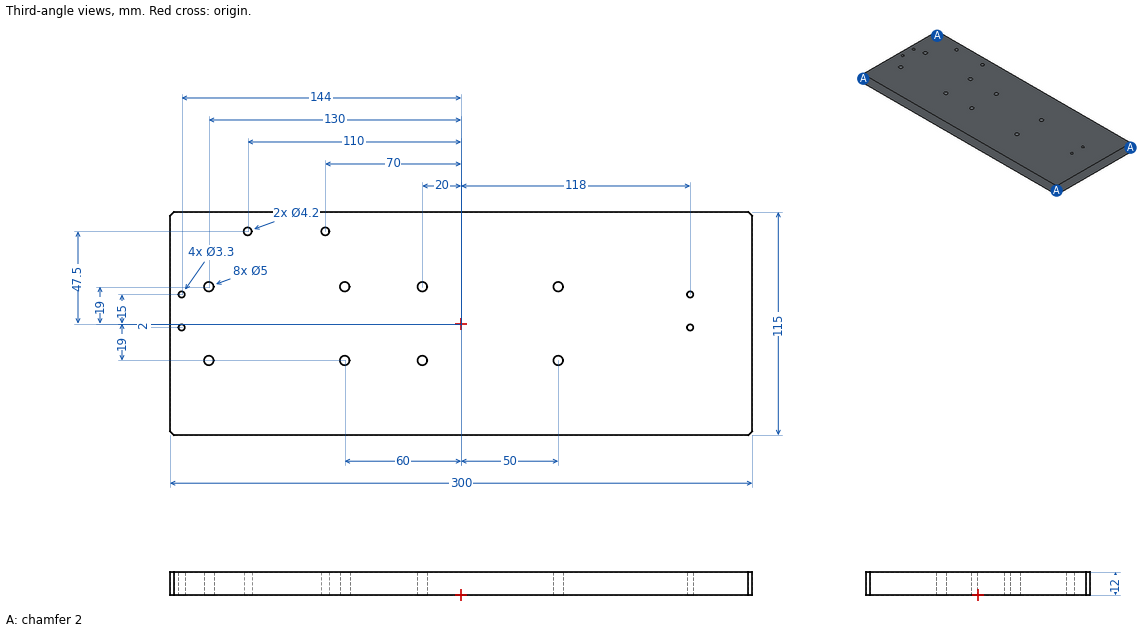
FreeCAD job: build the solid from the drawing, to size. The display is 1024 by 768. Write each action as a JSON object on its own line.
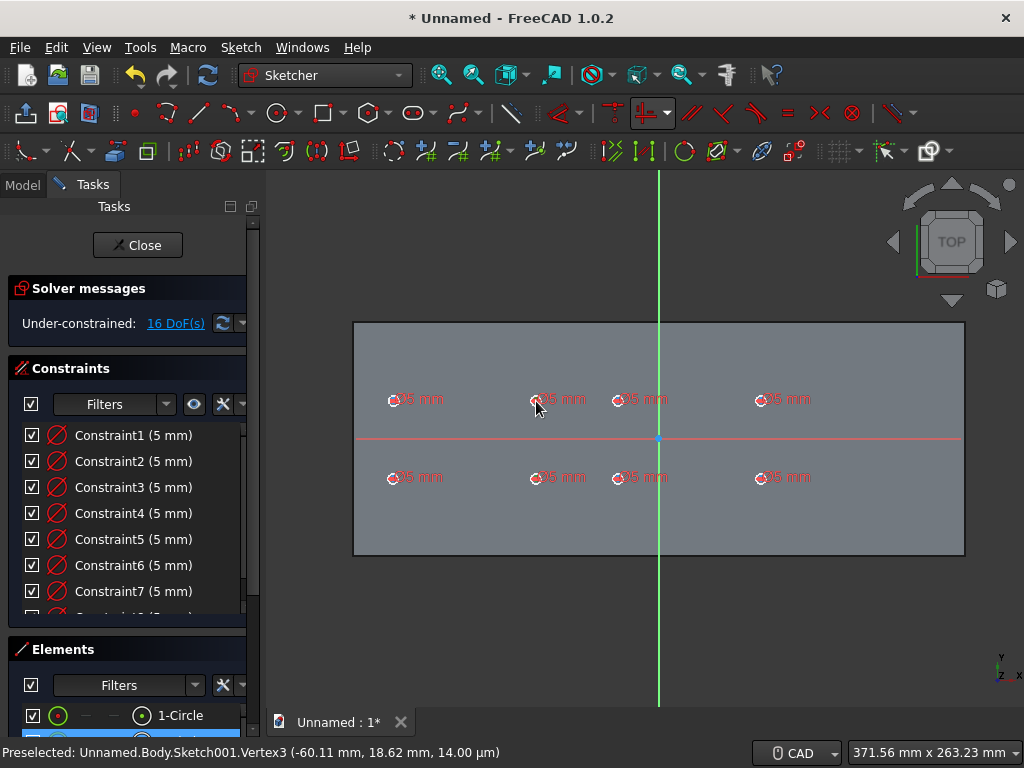
{"action": "left_click", "coordinate": [670, 114]}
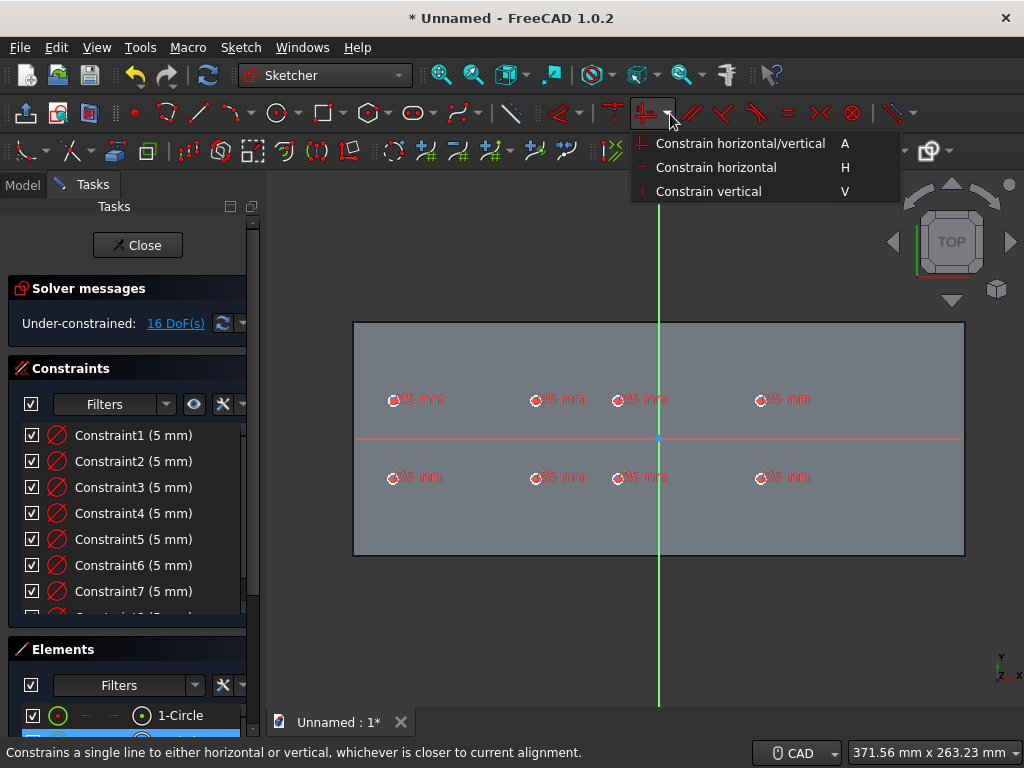
{"action": "left_click", "coordinate": [766, 191]}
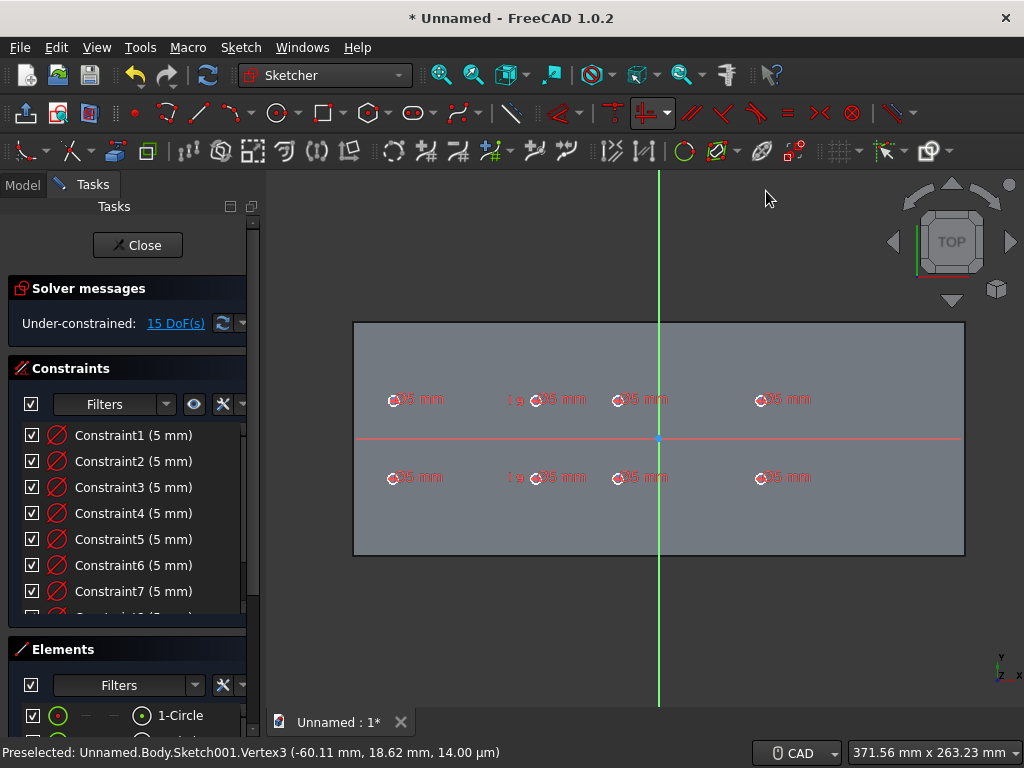
{"action": "left_click", "coordinate": [394, 401]}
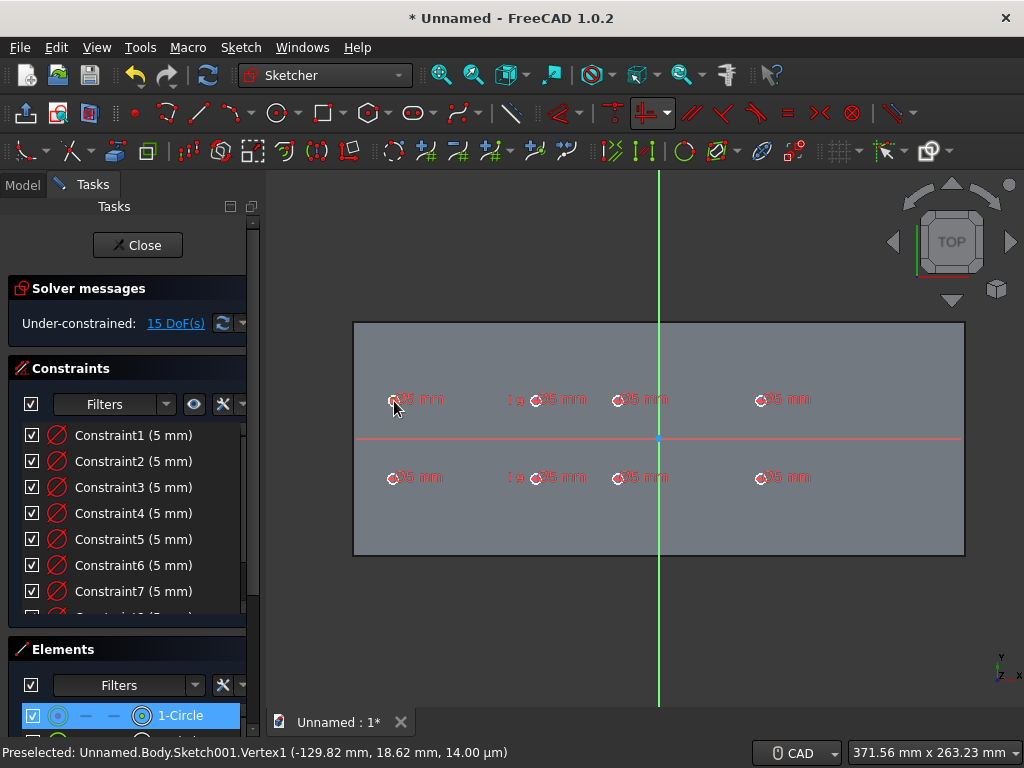
{"action": "left_click", "coordinate": [536, 401]}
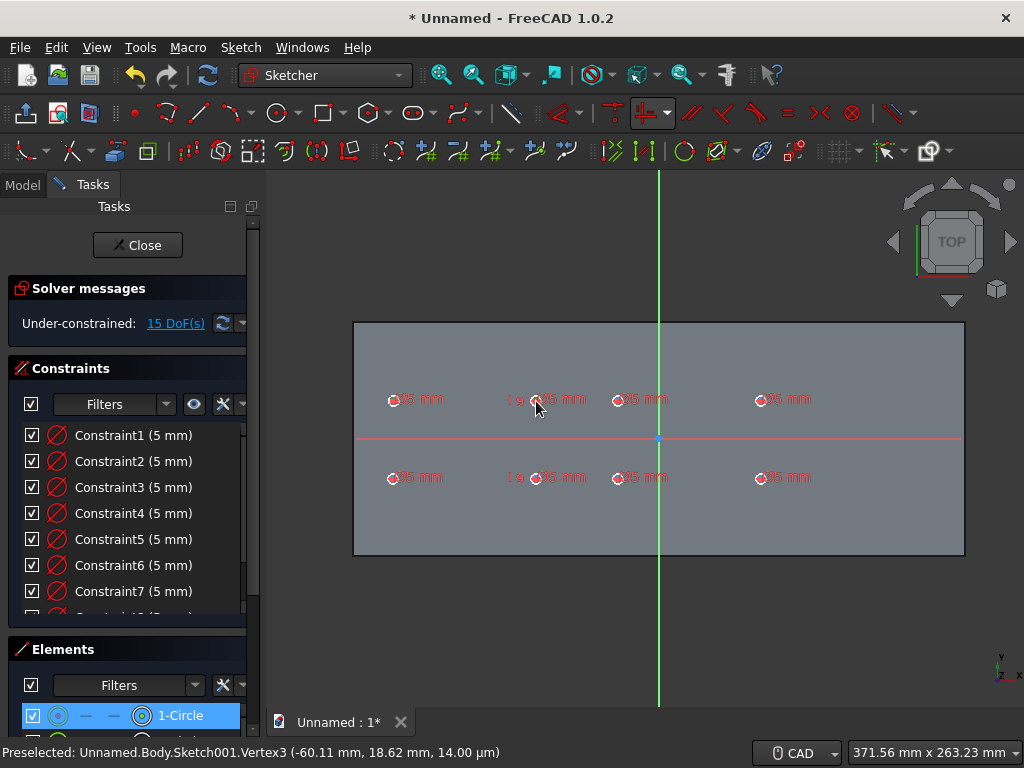
{"action": "left_click", "coordinate": [670, 114]}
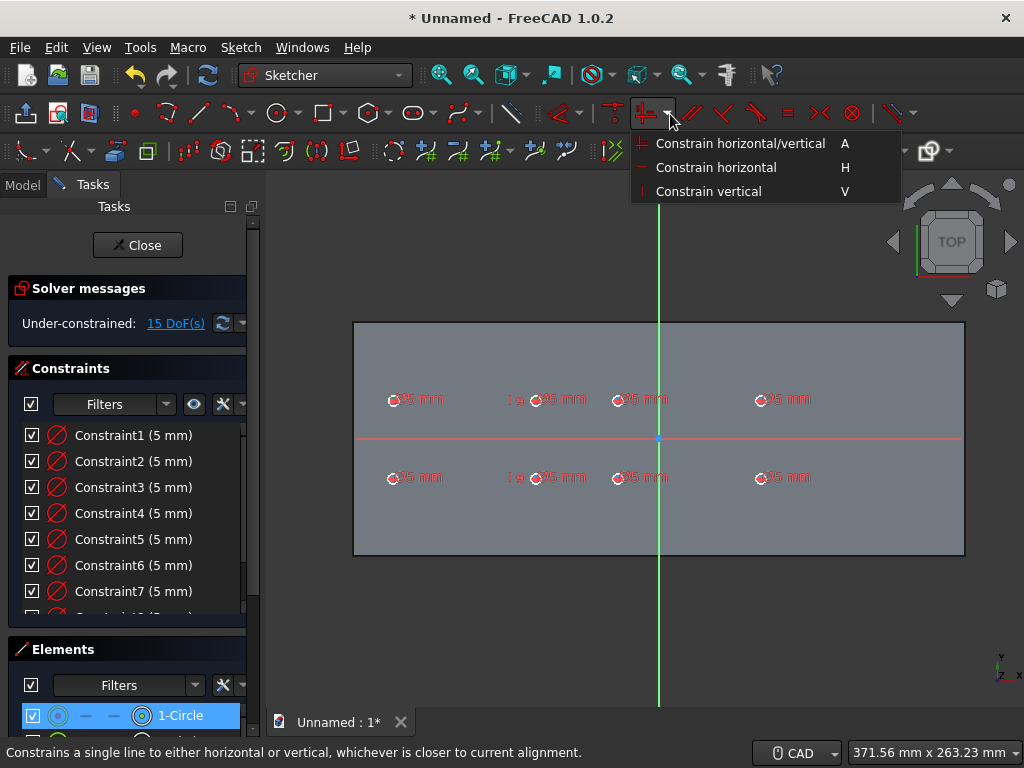
{"action": "left_click", "coordinate": [766, 167]}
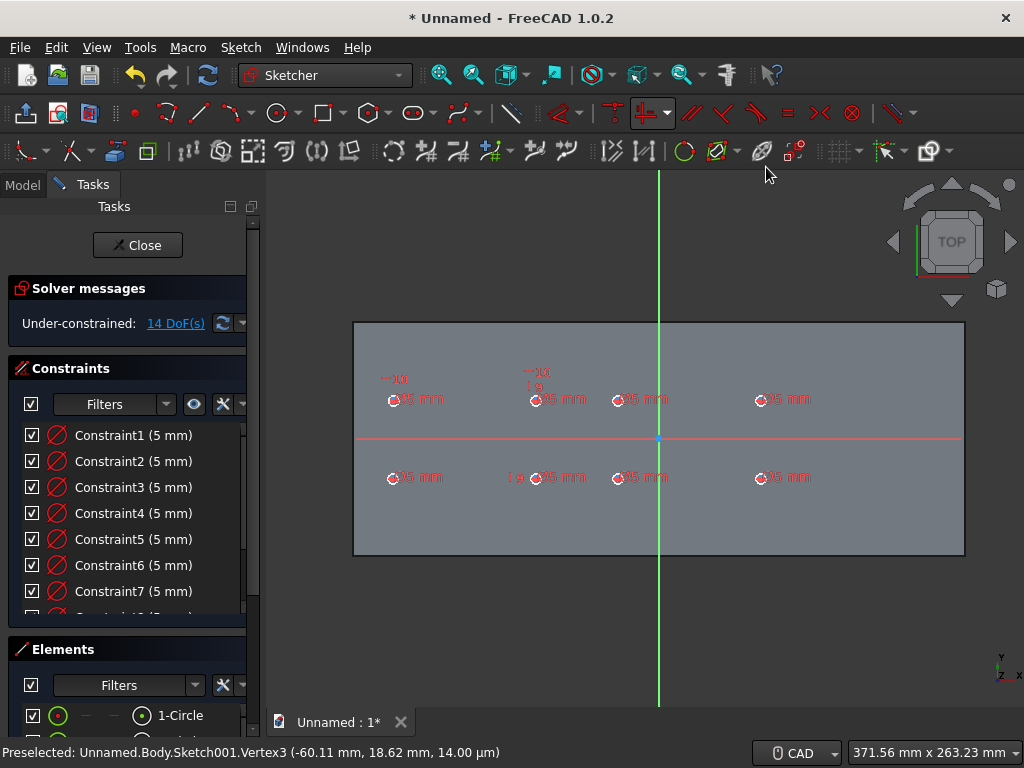
{"action": "left_click", "coordinate": [394, 401]}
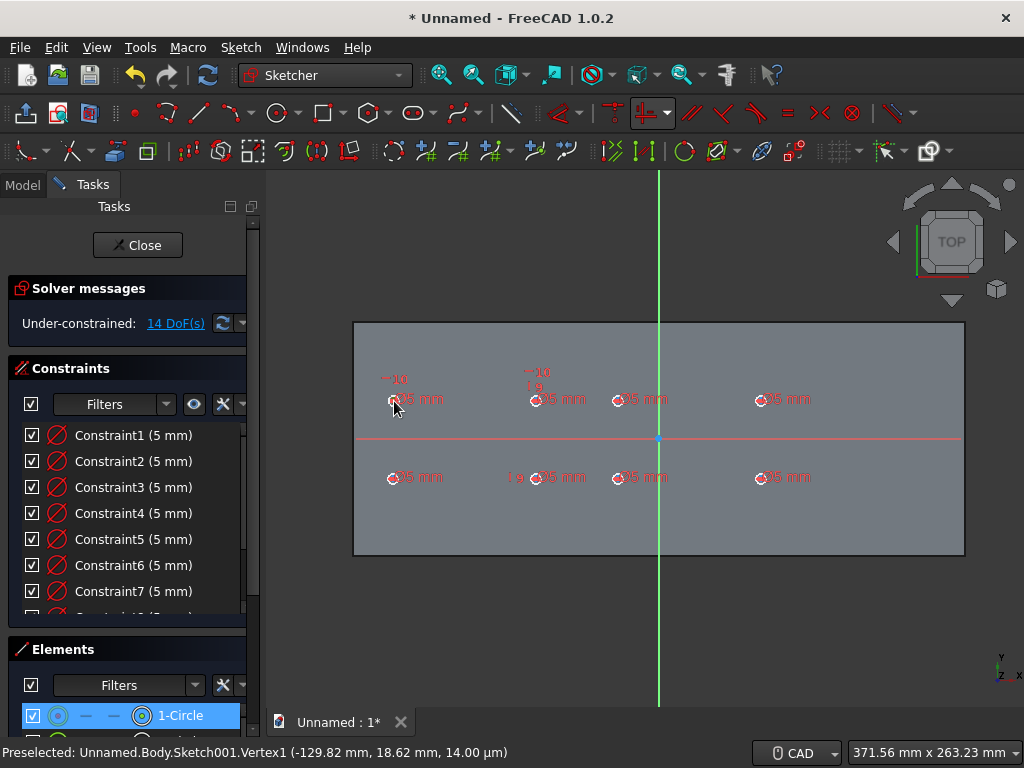
{"action": "left_click", "coordinate": [393, 479]}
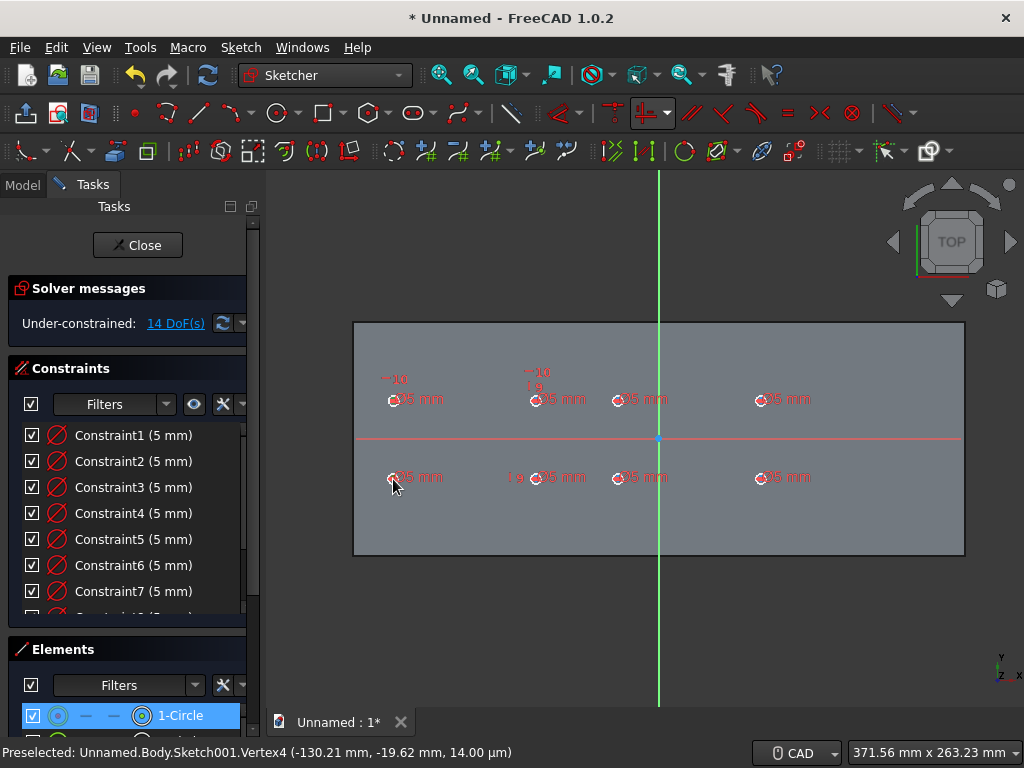
{"action": "key", "text": "v"}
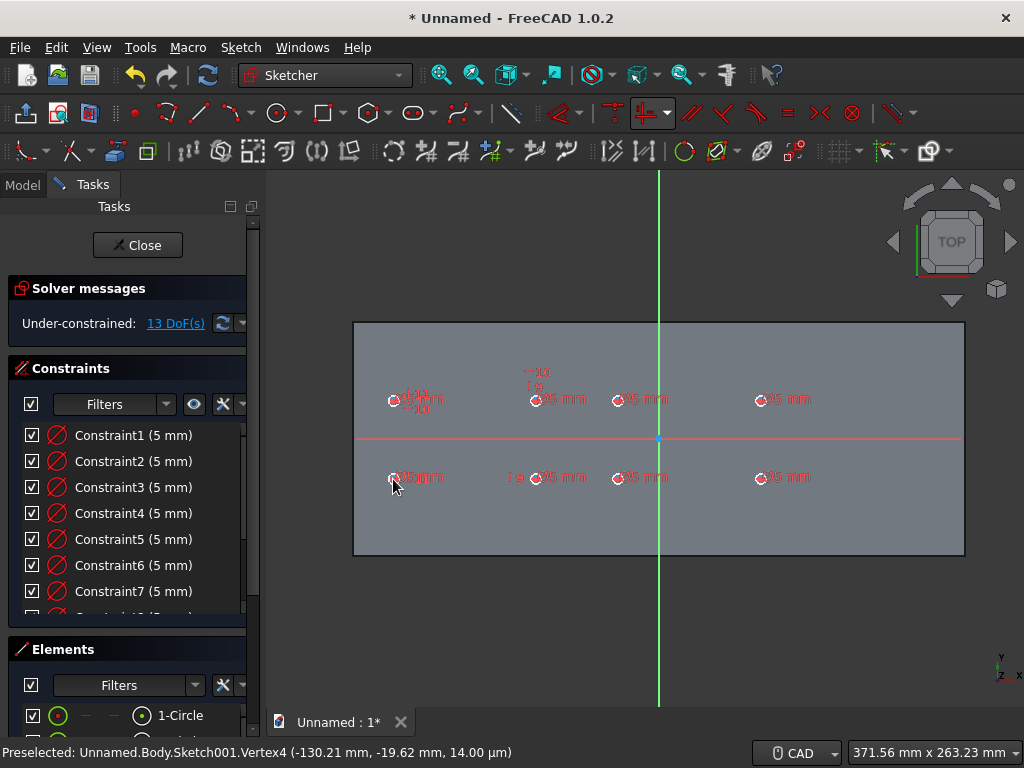
{"action": "left_click", "coordinate": [536, 479]}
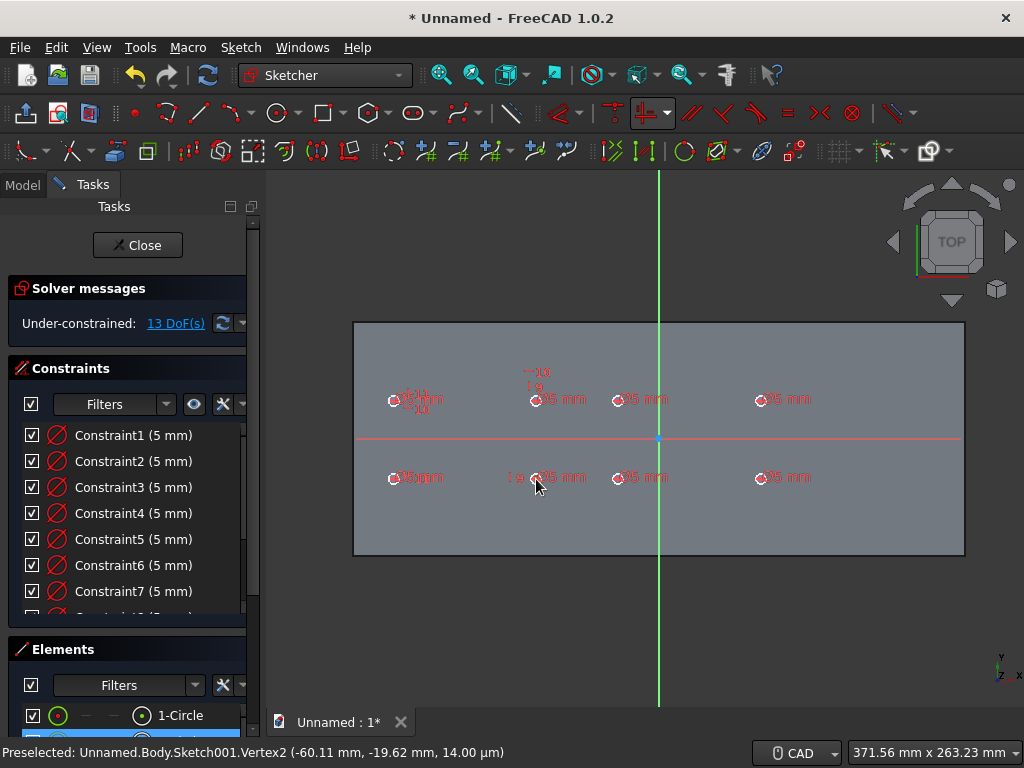
{"action": "left_click", "coordinate": [394, 479]}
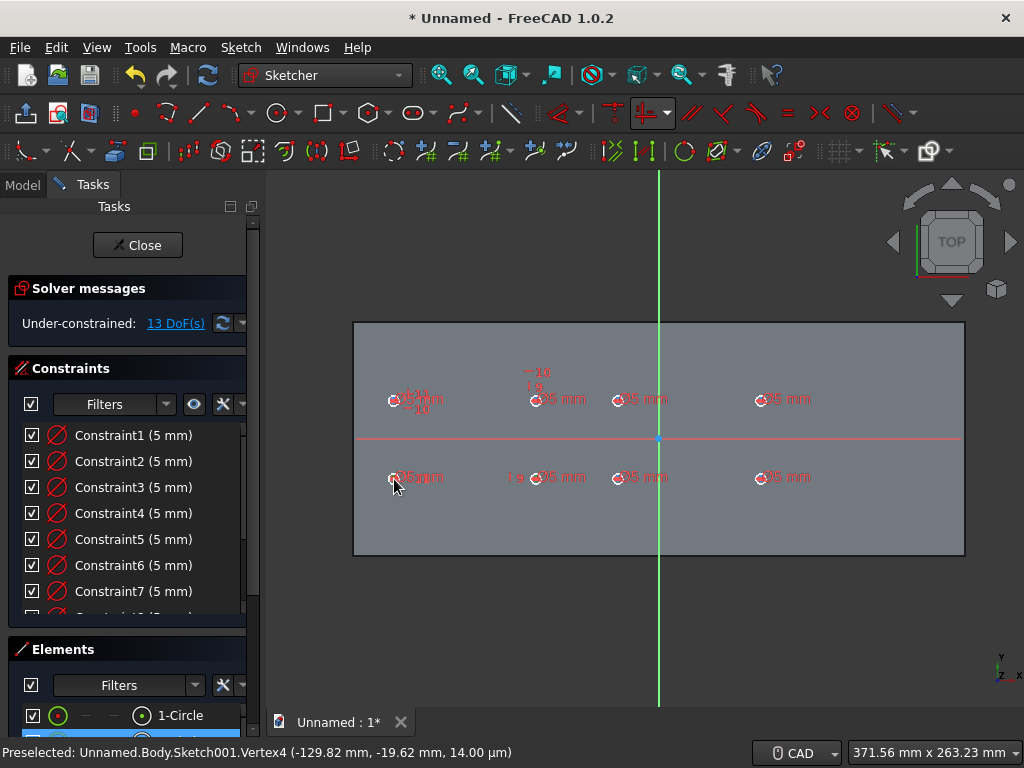
{"action": "key", "text": "h"}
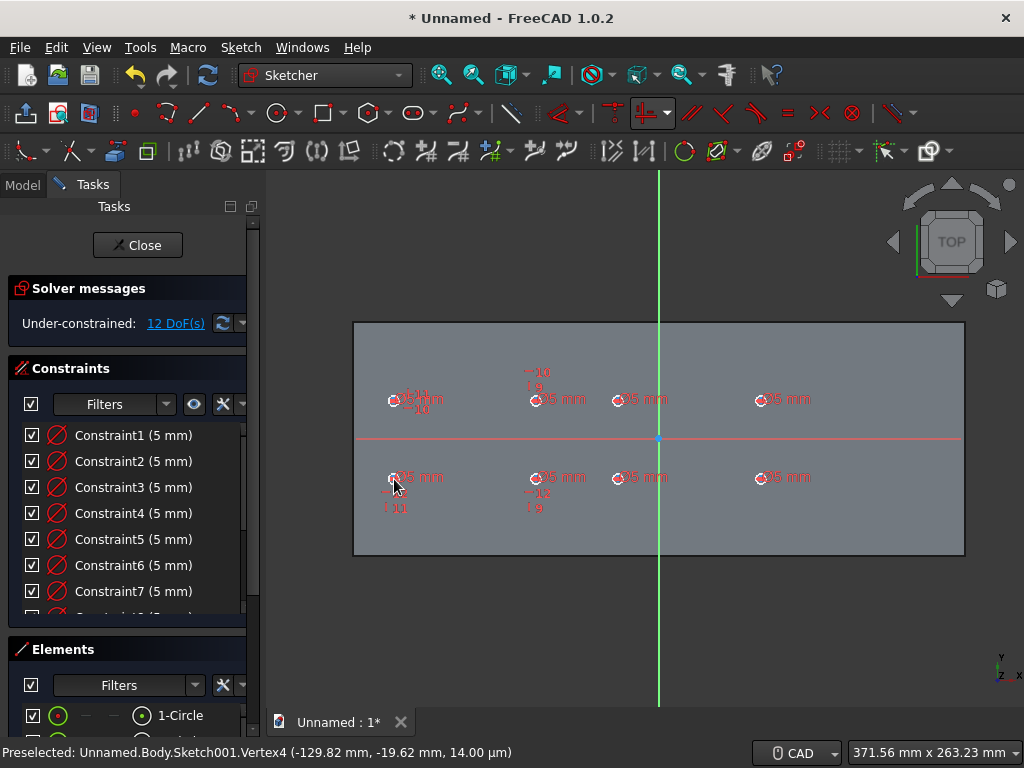
{"action": "left_click", "coordinate": [536, 401]}